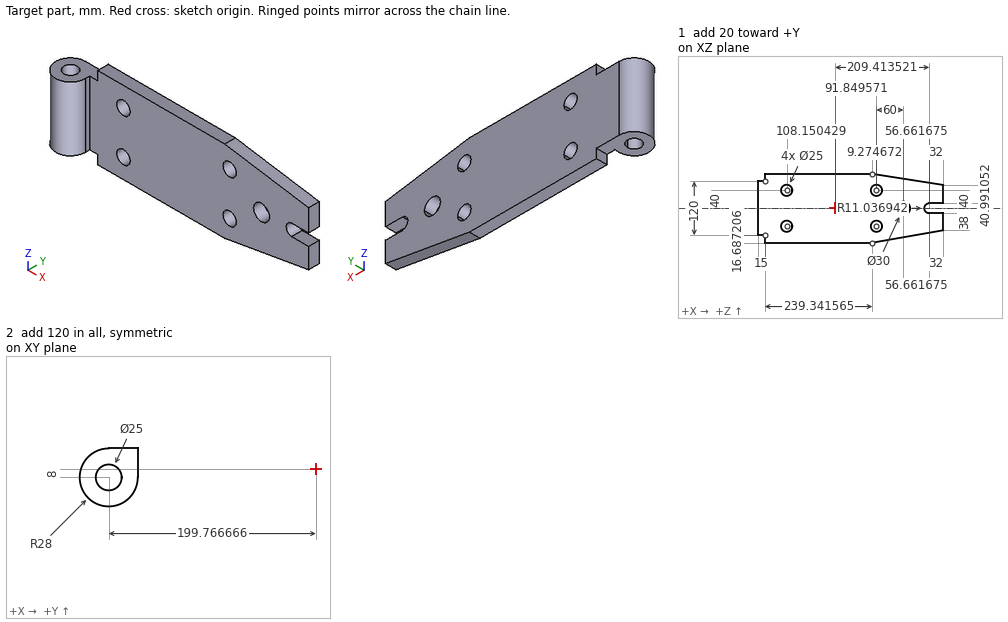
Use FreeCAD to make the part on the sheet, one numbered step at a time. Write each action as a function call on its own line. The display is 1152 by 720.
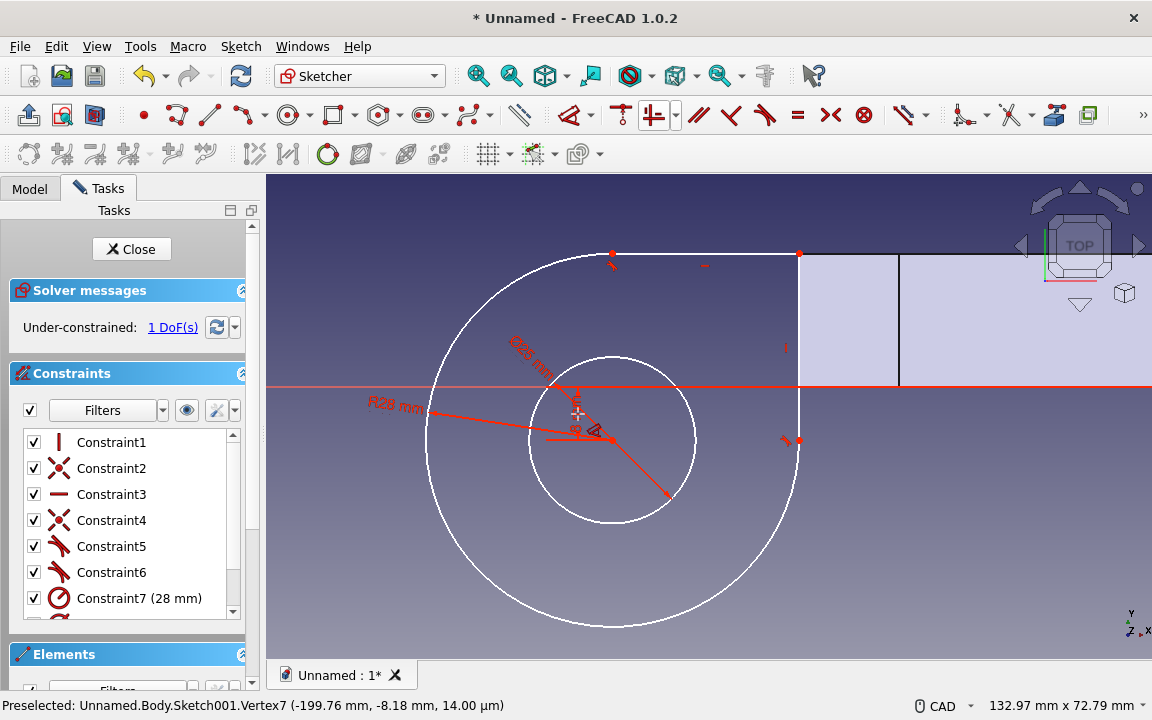
click(612, 440)
click(714, 474)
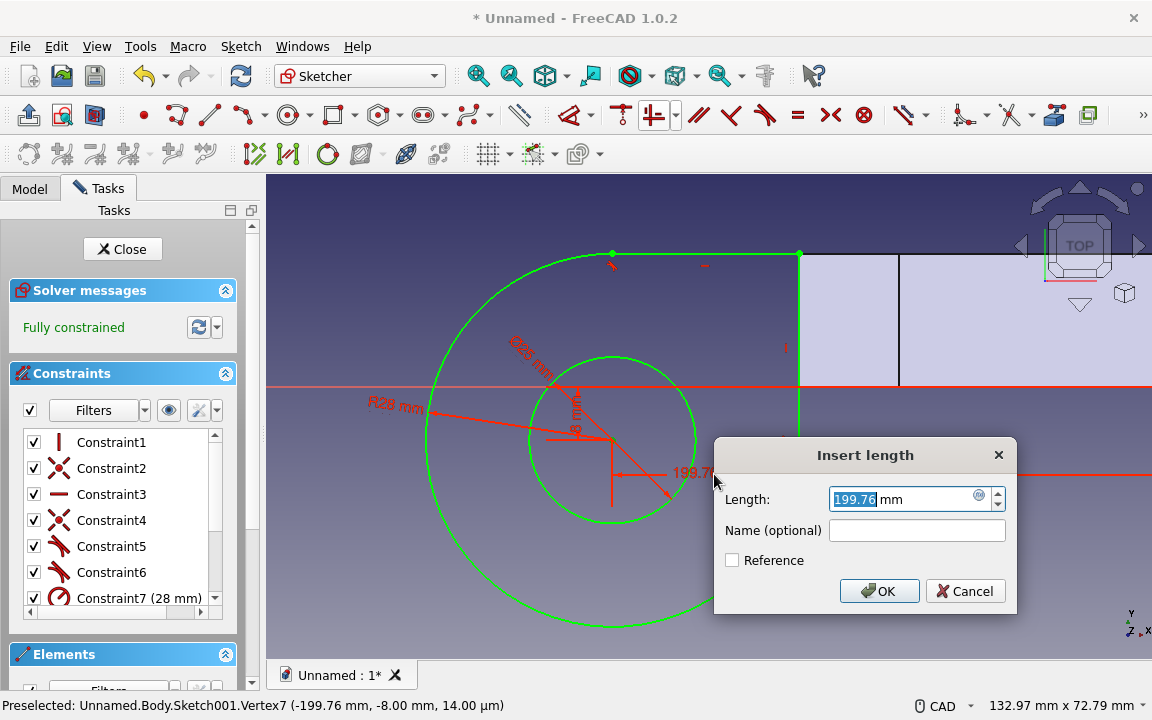
text(199.766666)
key(Return)
key(Escape)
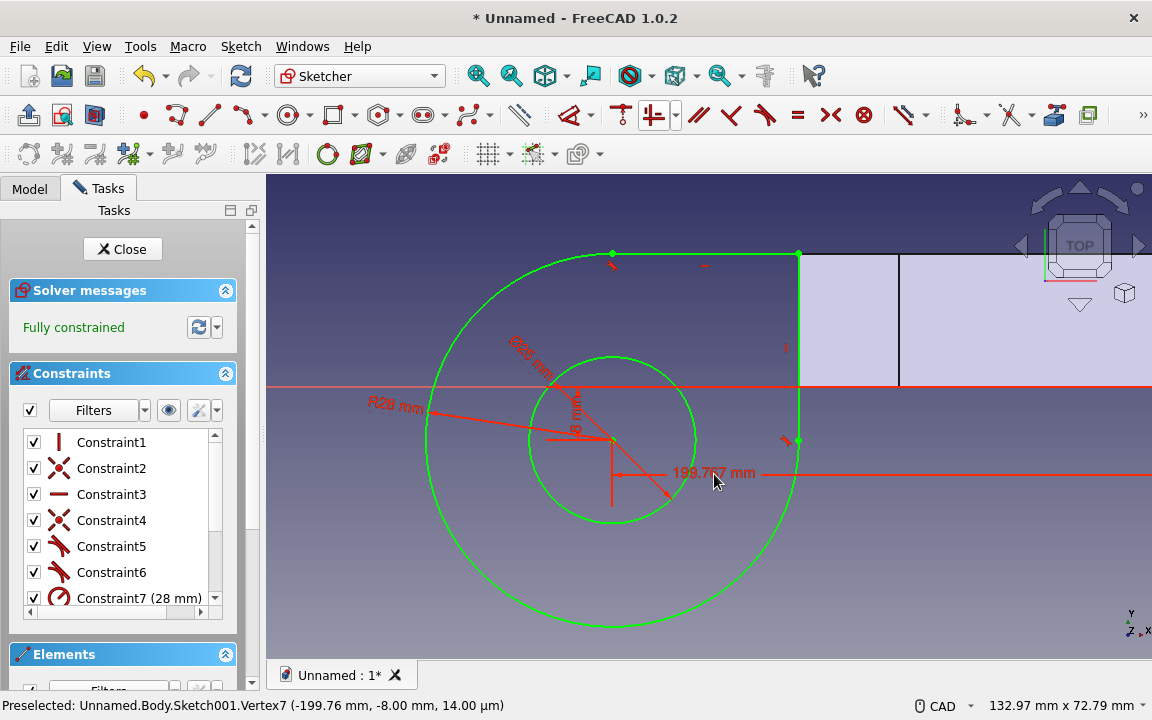
click(123, 249)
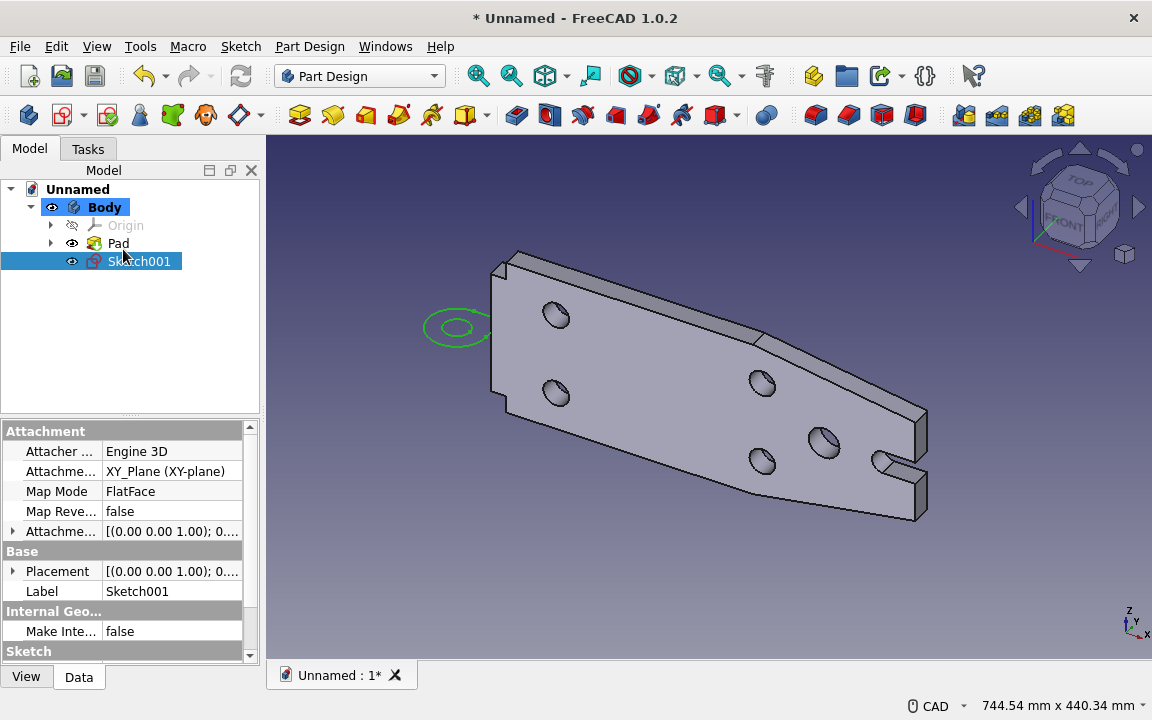
click(300, 116)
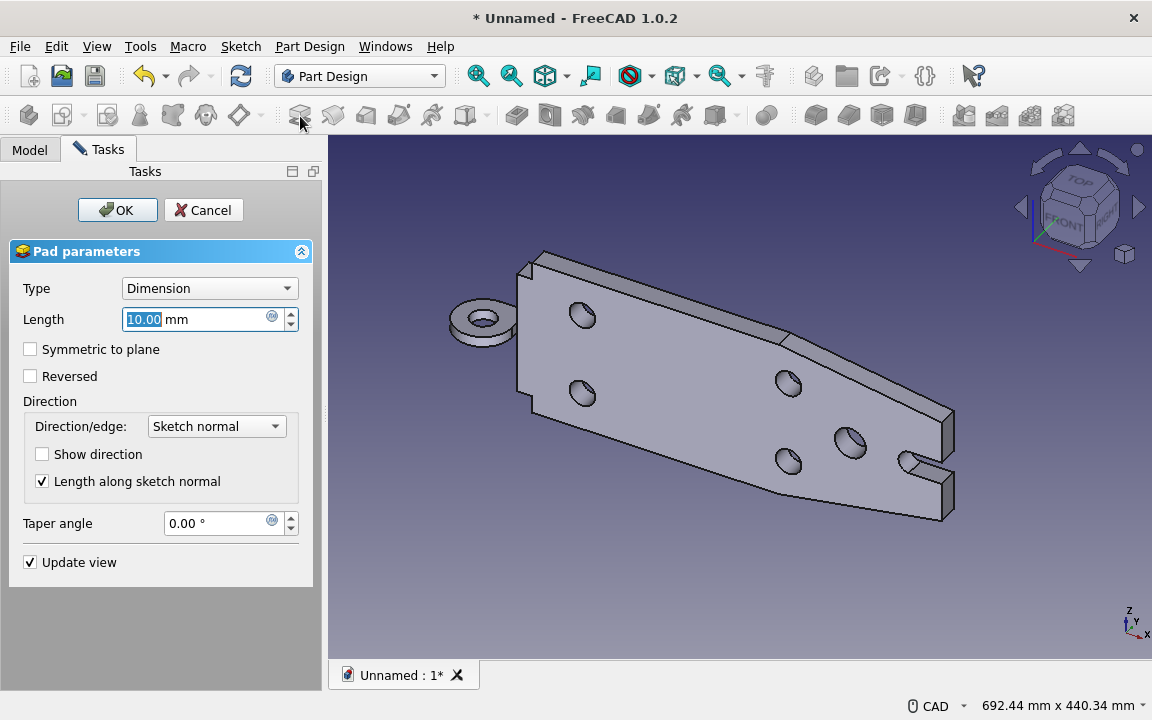
text(120)
key(Tab)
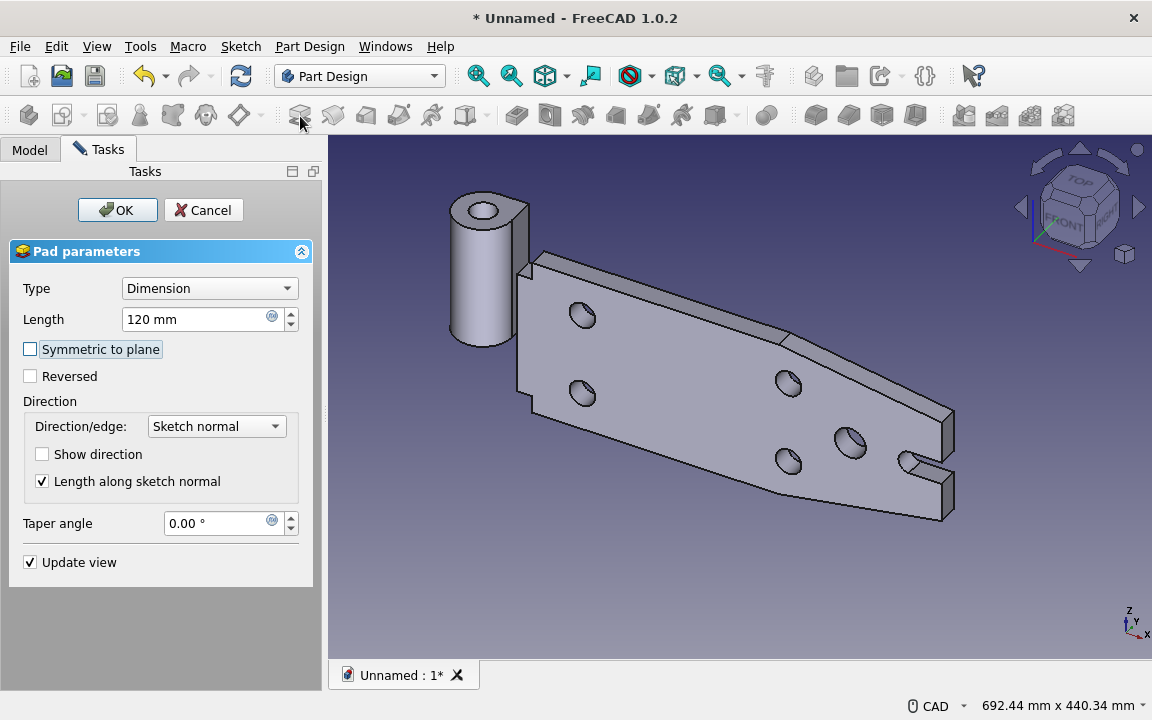
click(31, 349)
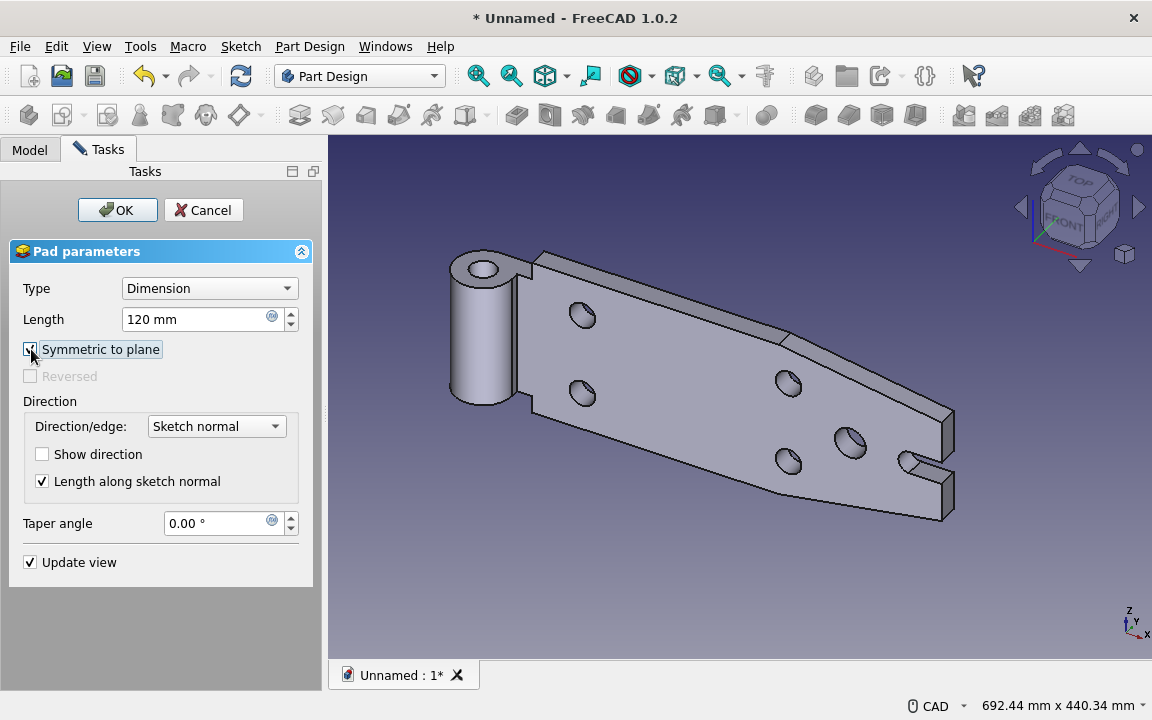
click(118, 210)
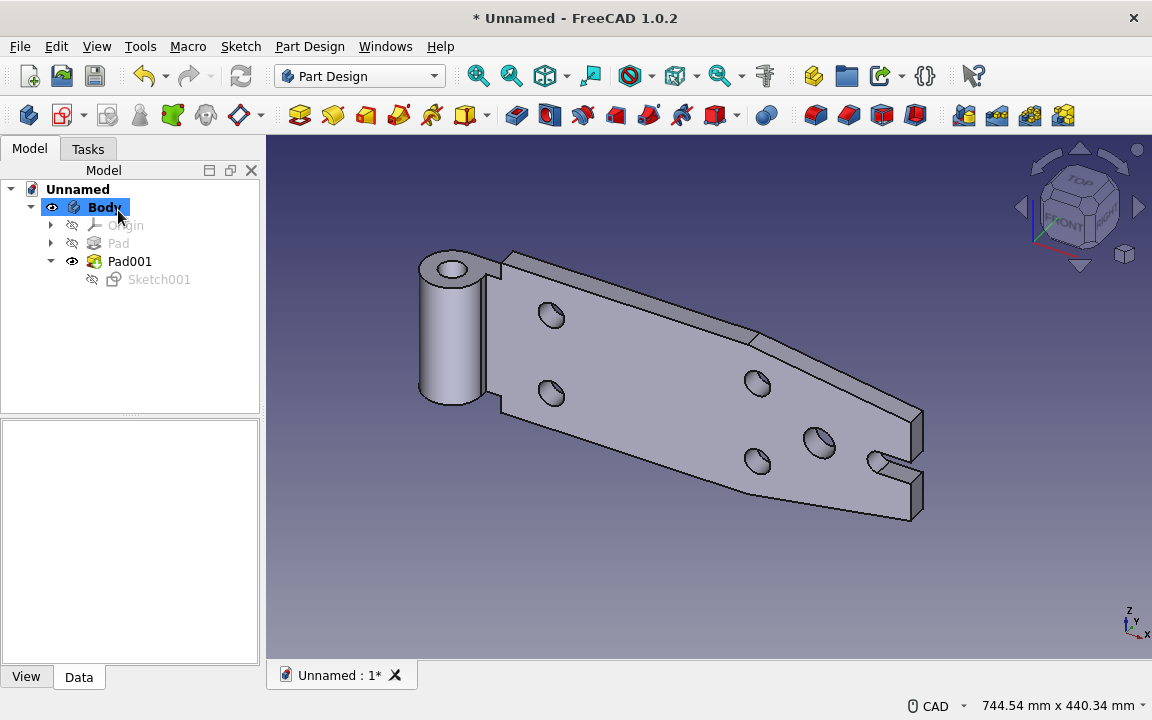
key(0)